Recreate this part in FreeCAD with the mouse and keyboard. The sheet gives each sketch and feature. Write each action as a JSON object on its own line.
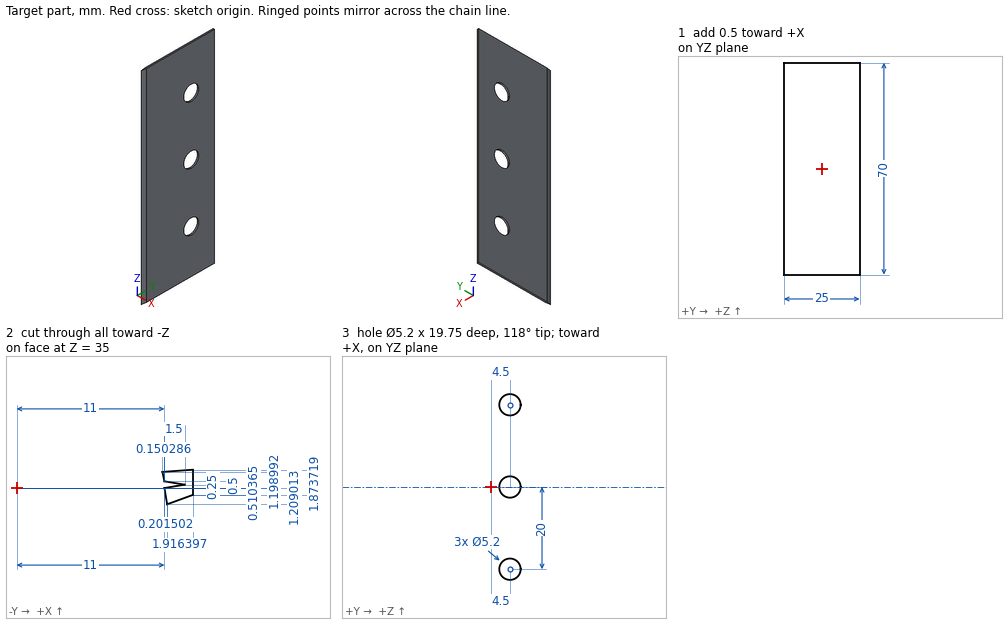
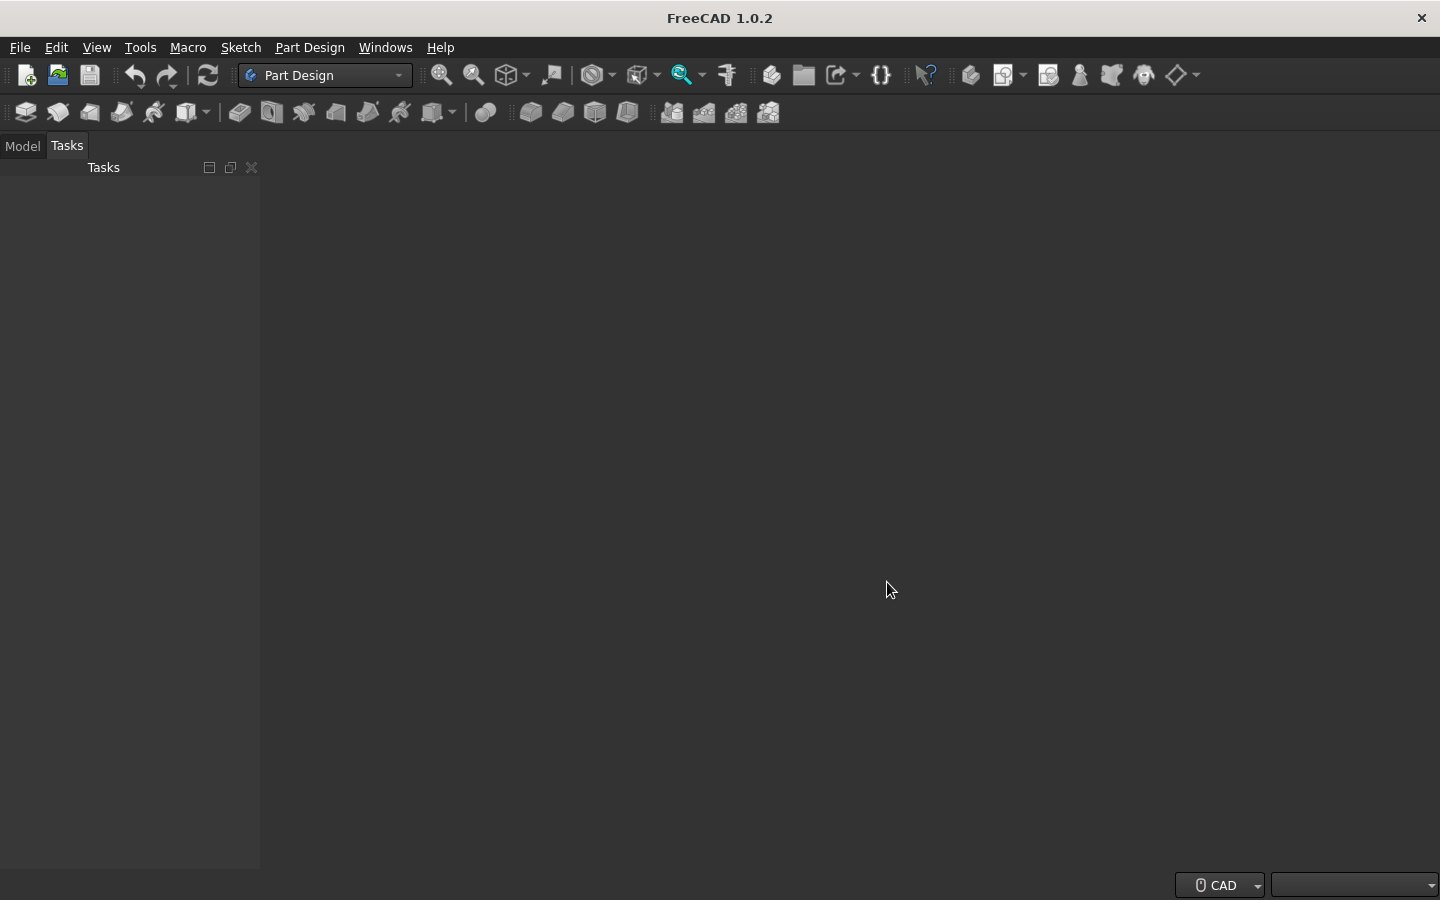
{"action": "left_click", "coordinate": [26, 76]}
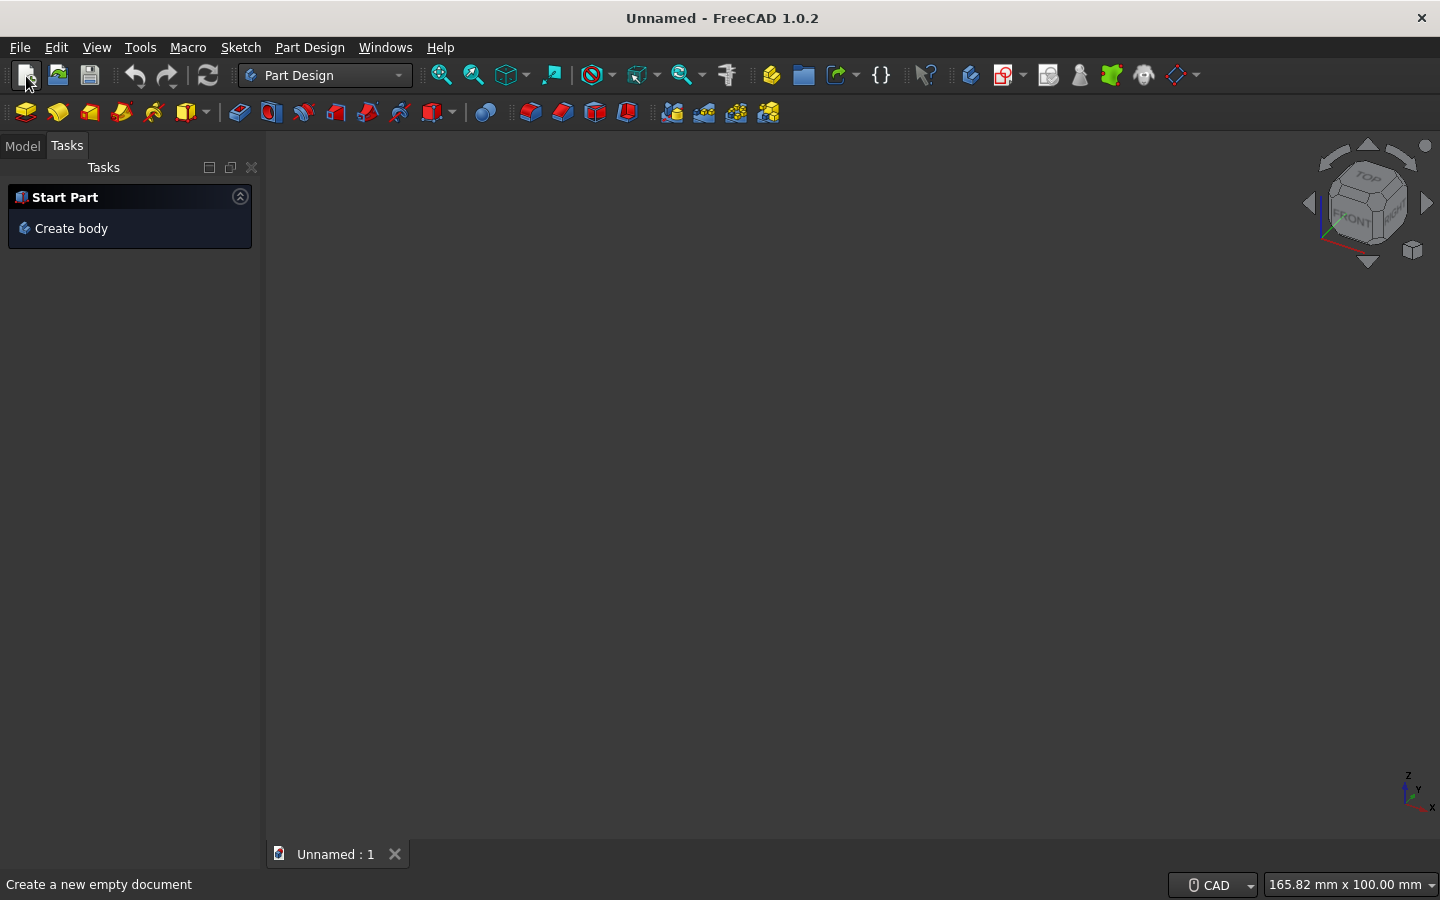
{"action": "left_click", "coordinate": [1004, 76]}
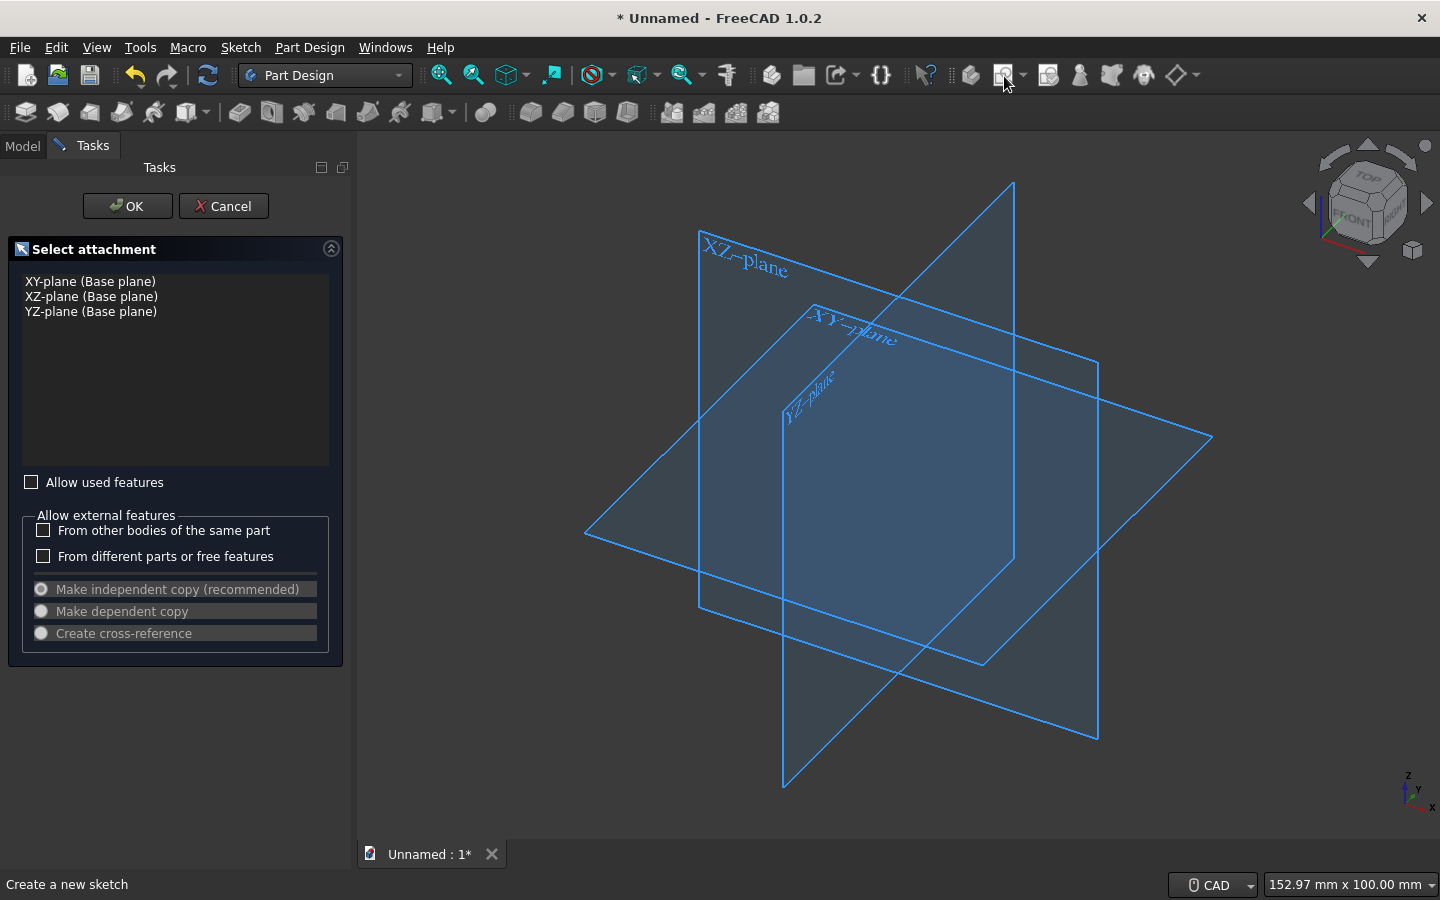
{"action": "left_click", "coordinate": [82, 312]}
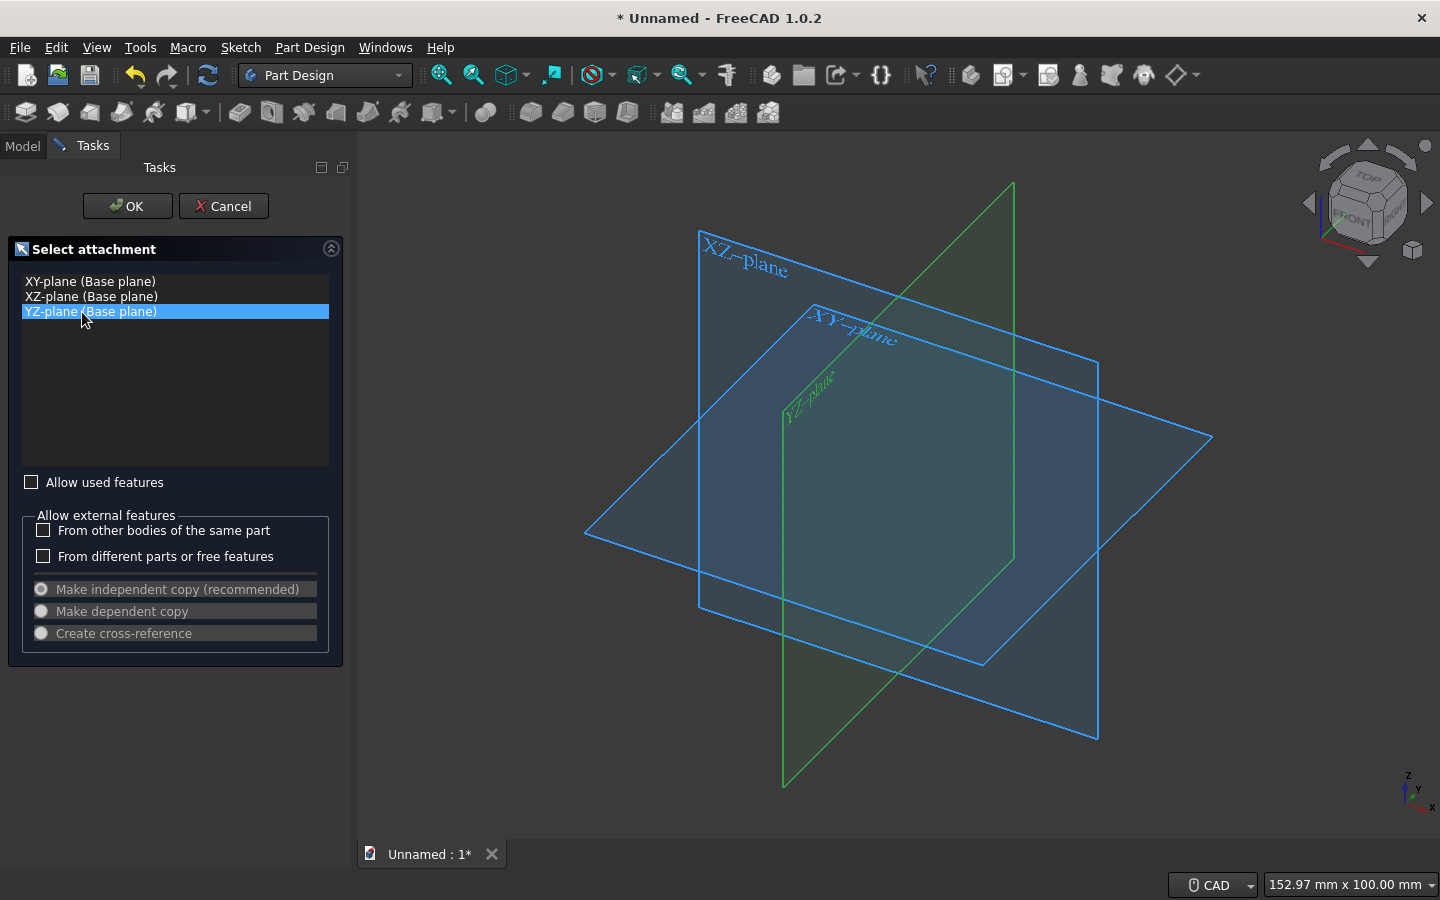
{"action": "left_click", "coordinate": [128, 206]}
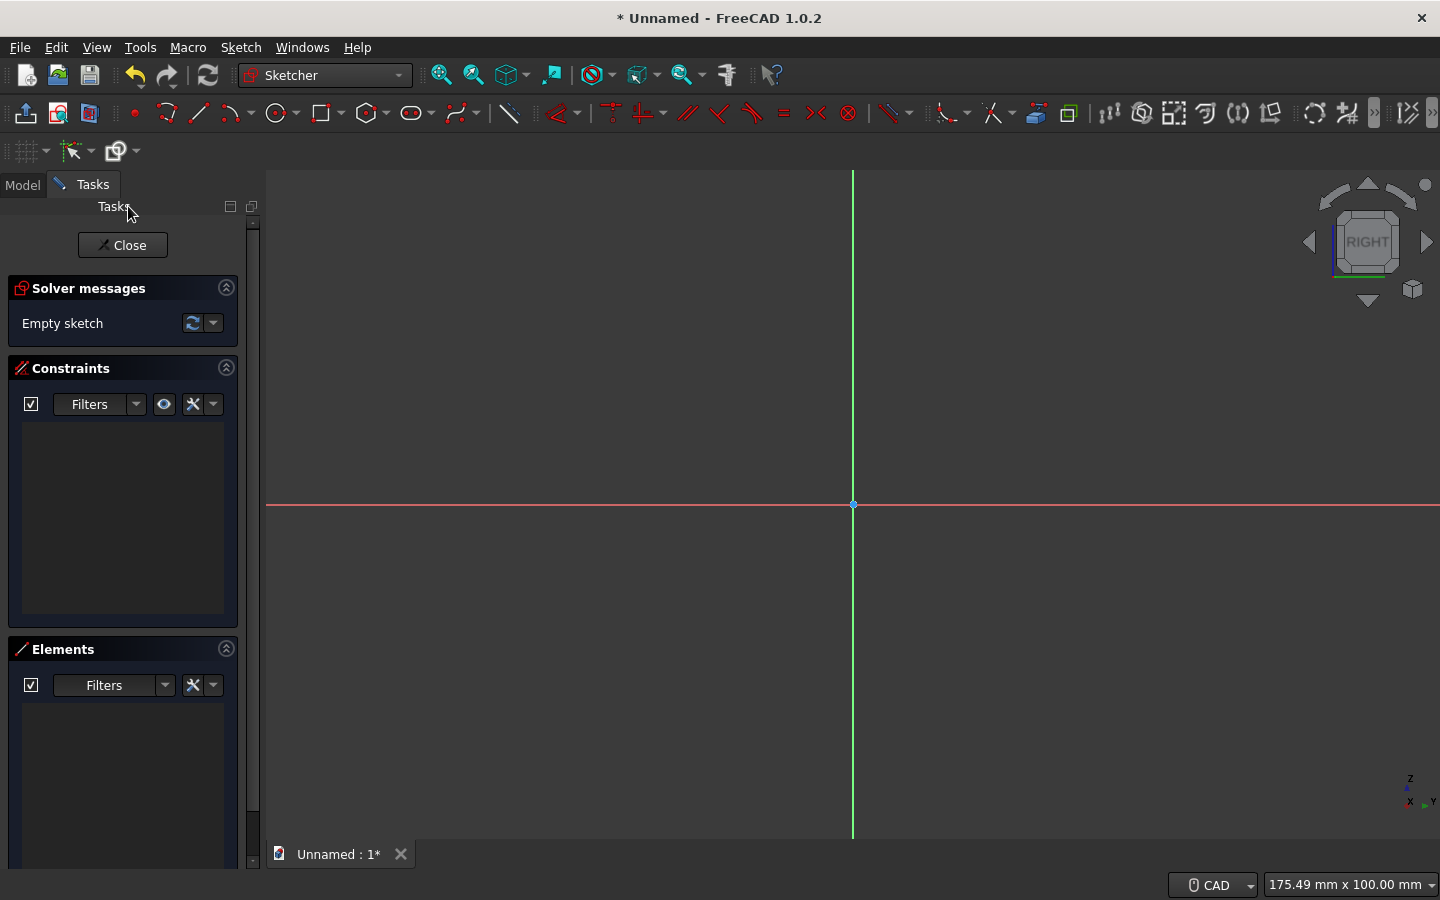
{"action": "key", "text": "g v"}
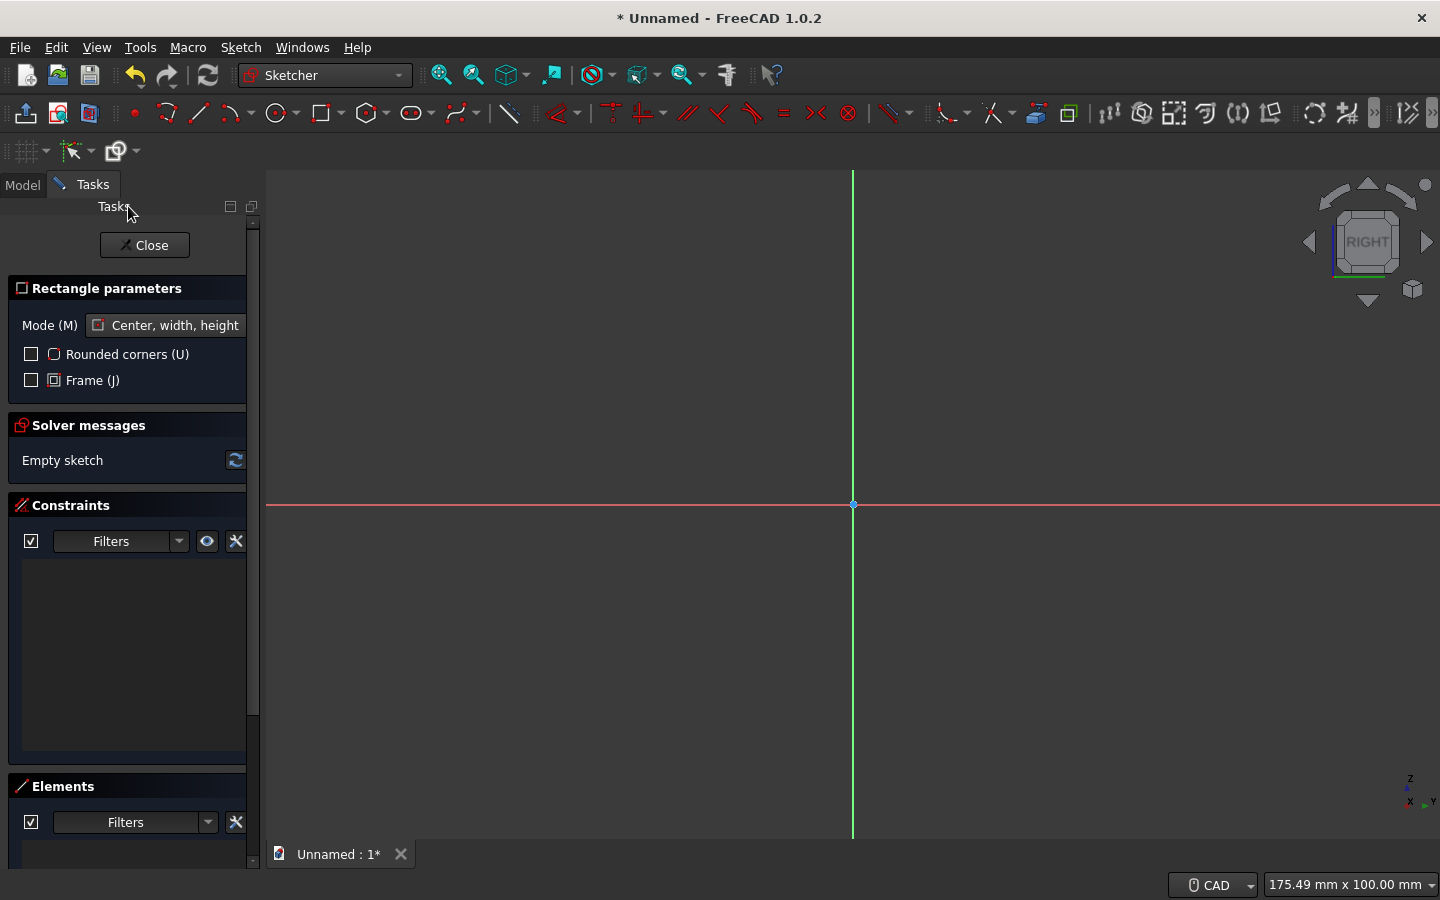
{"action": "left_click", "coordinate": [853, 504]}
{"action": "mouse_move", "coordinate": [937, 270]}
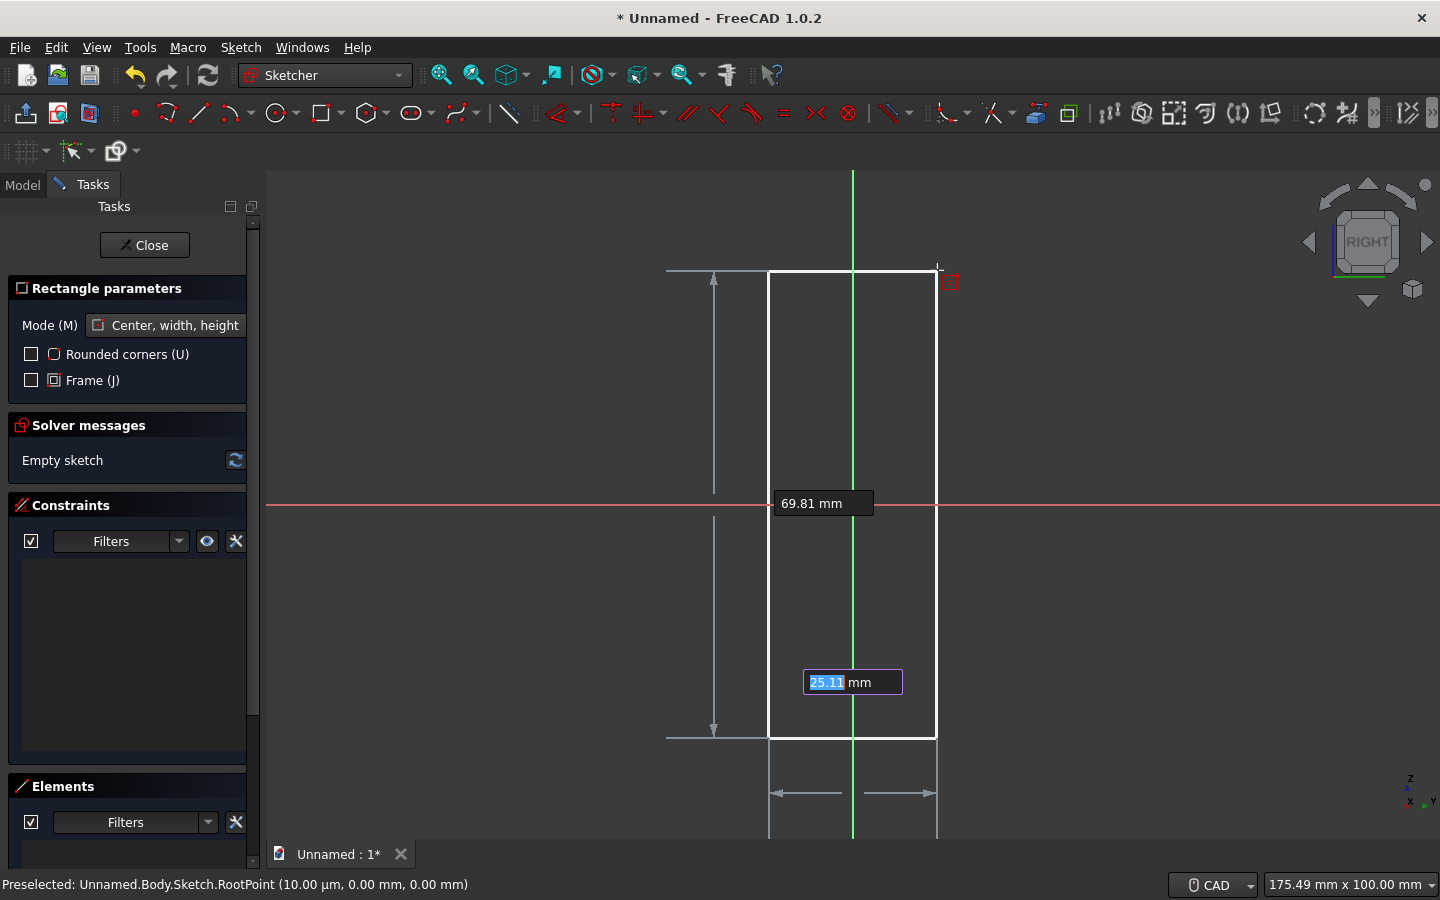
{"action": "type", "text": "25"}
{"action": "key", "text": "Tab"}
{"action": "type", "text": "70"}
{"action": "key", "text": "Return"}
{"action": "key", "text": "Escape"}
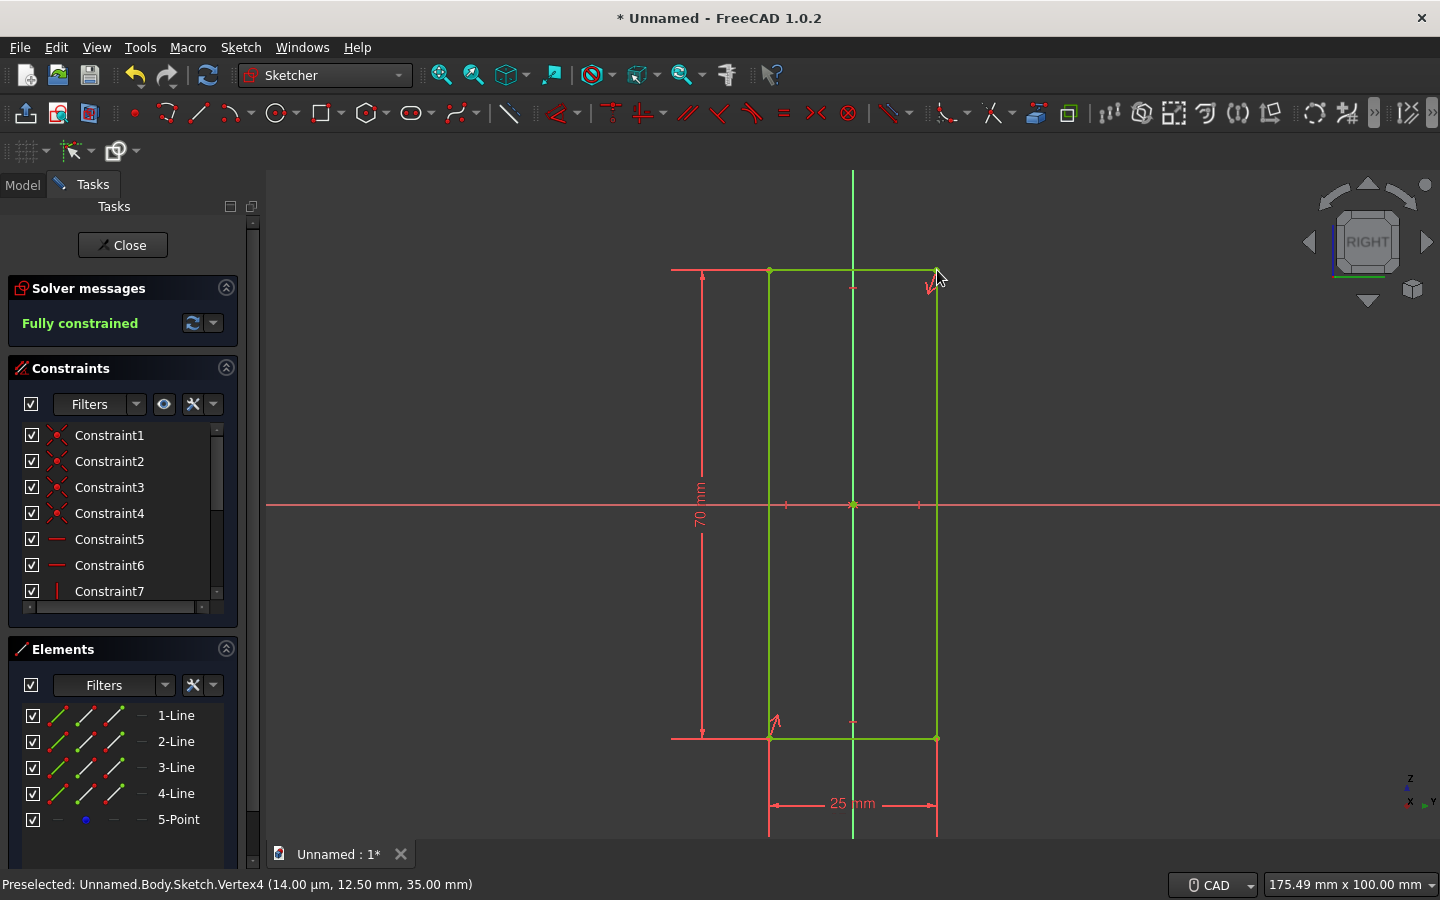
{"action": "left_click", "coordinate": [123, 245]}